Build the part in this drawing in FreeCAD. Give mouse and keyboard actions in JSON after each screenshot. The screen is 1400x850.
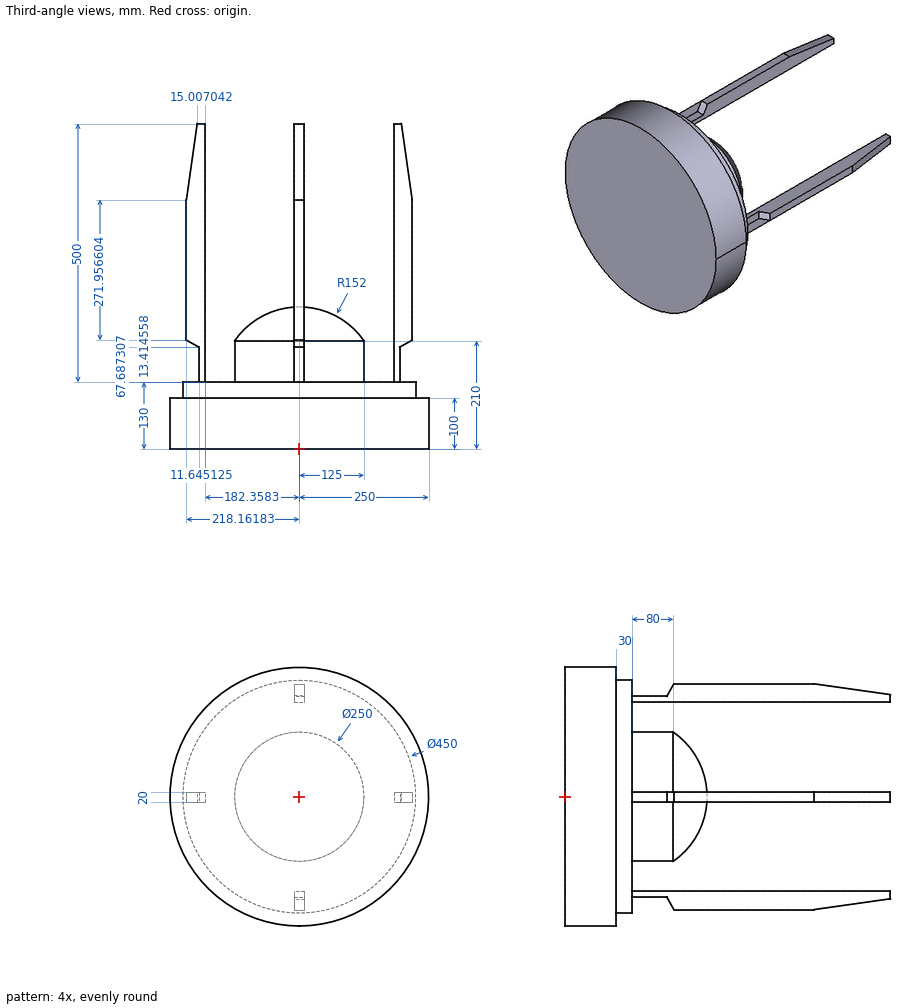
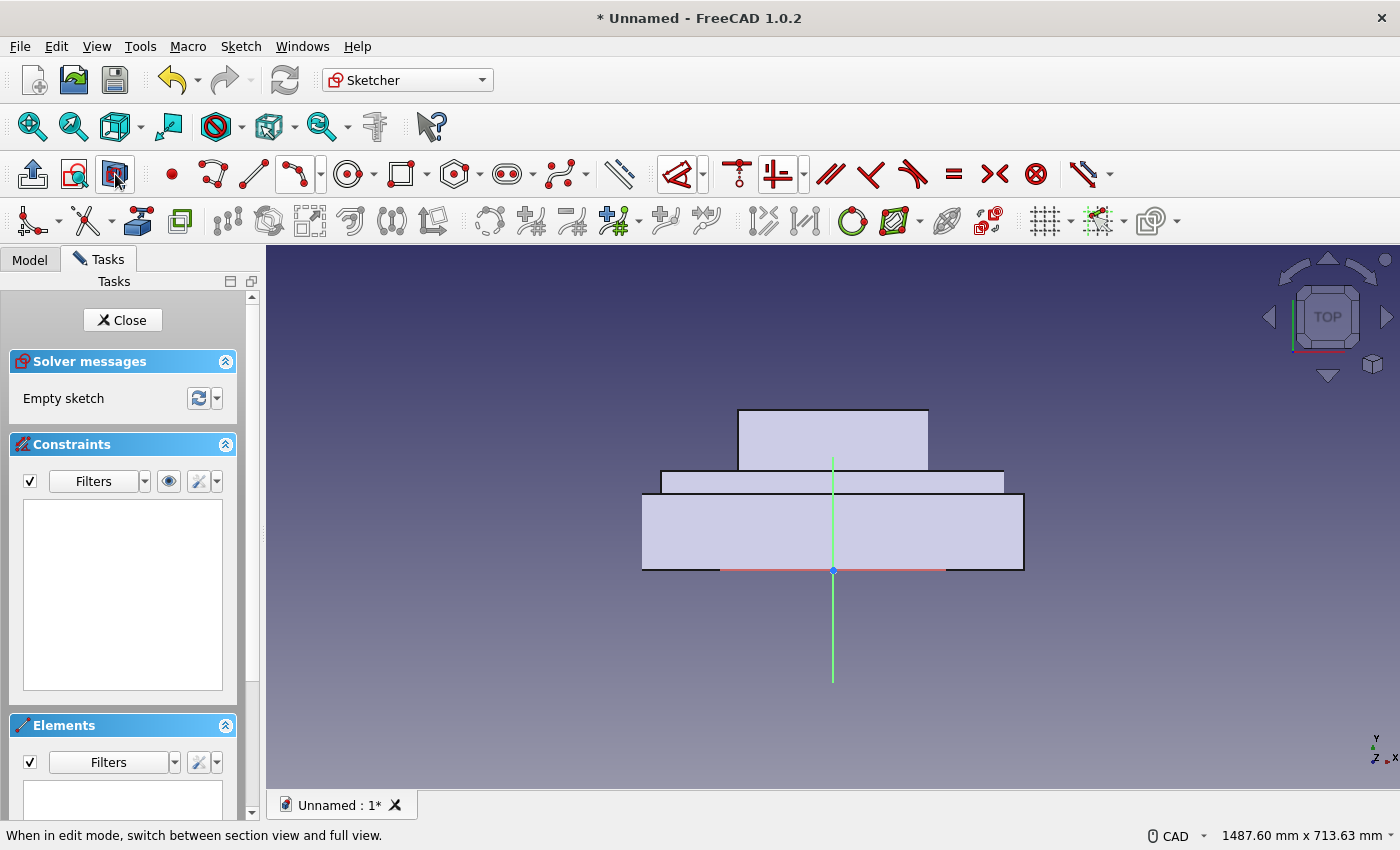
{"action": "scroll", "coordinate": [1117, 360], "scroll_direction": "up", "scroll_amount": 2}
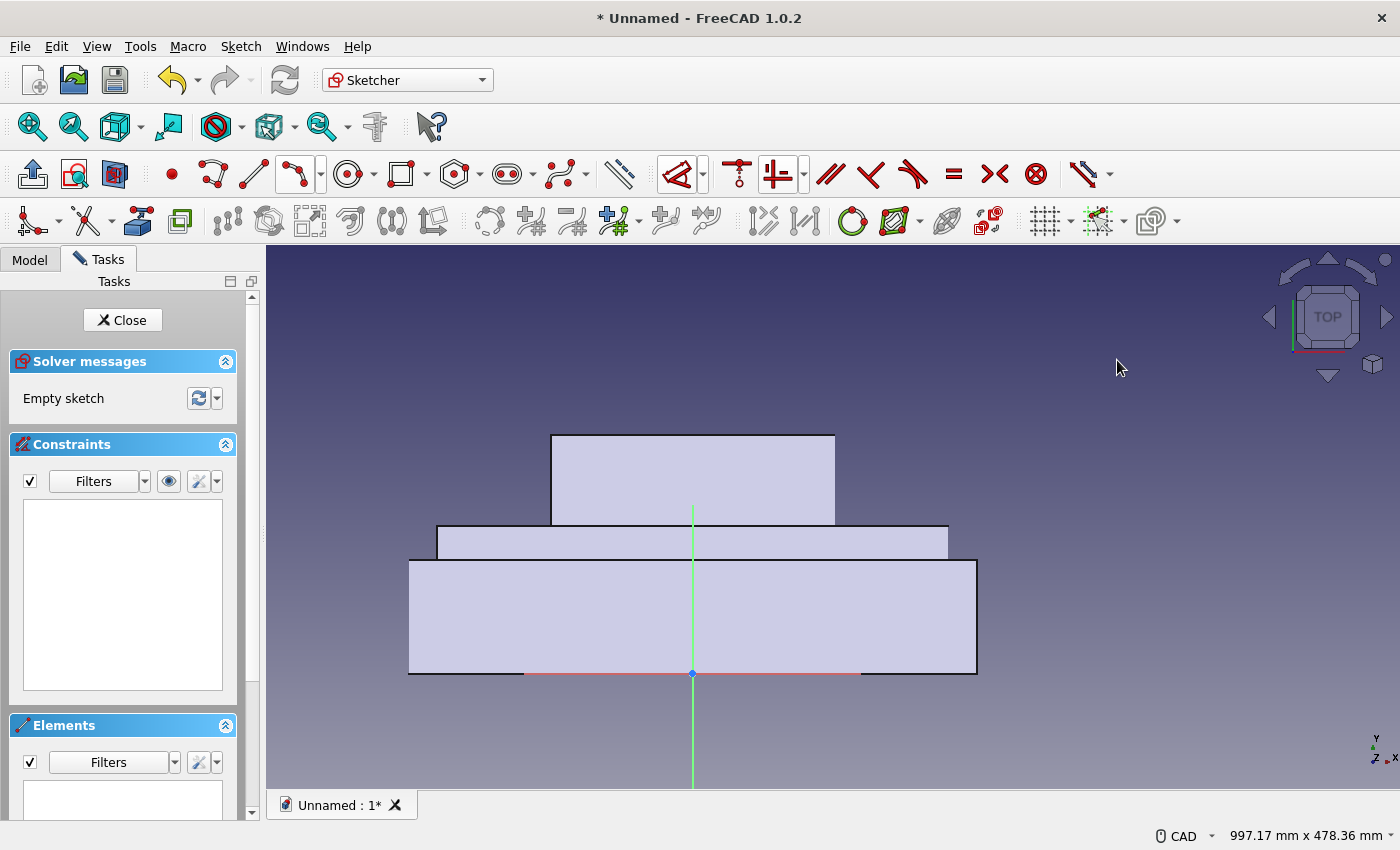
{"action": "left_click", "coordinate": [213, 174]}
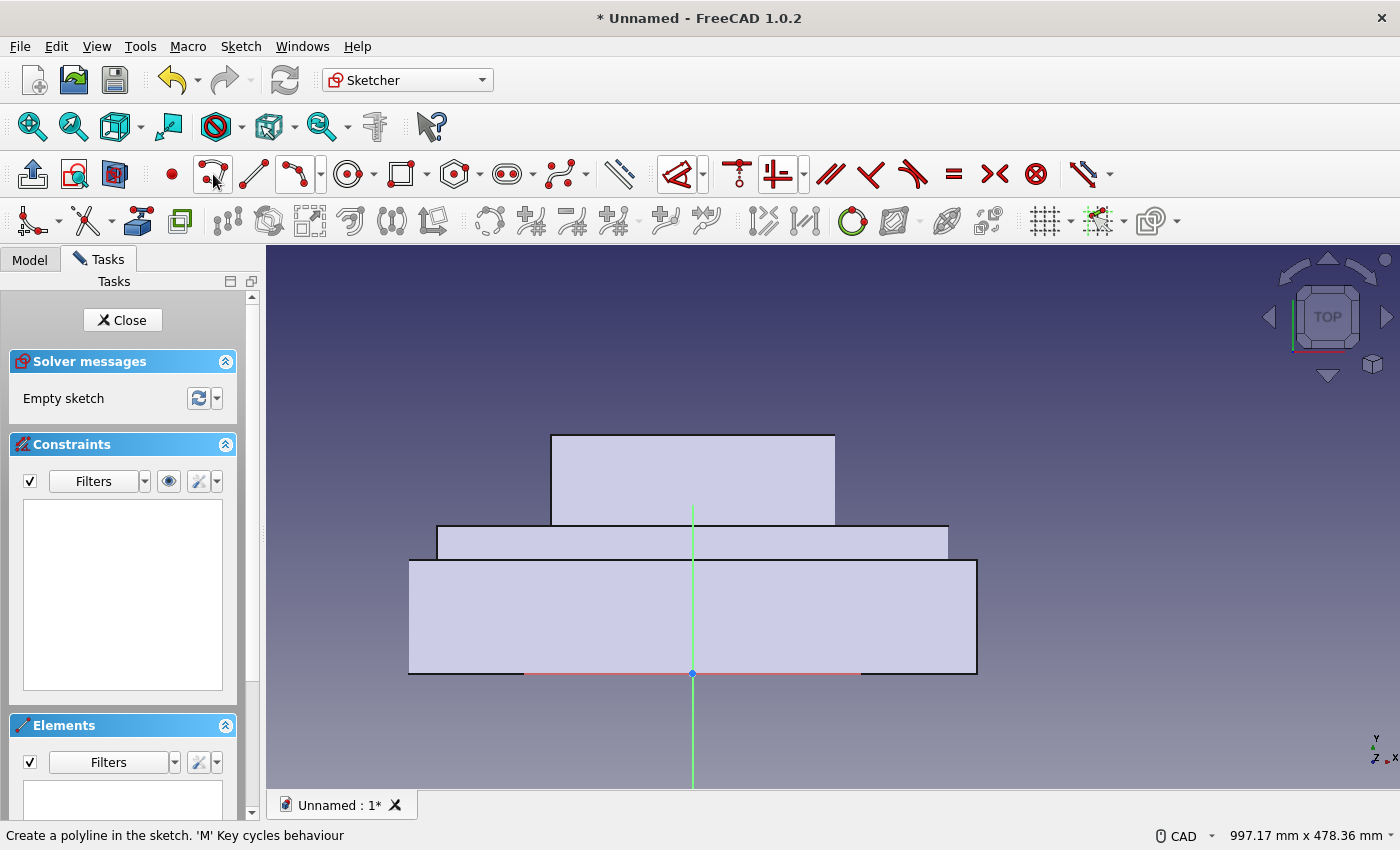
{"action": "left_click", "coordinate": [693, 360]}
{"action": "left_click", "coordinate": [702, 435]}
{"action": "left_click", "coordinate": [835, 435]}
{"action": "right_click", "coordinate": [835, 435]}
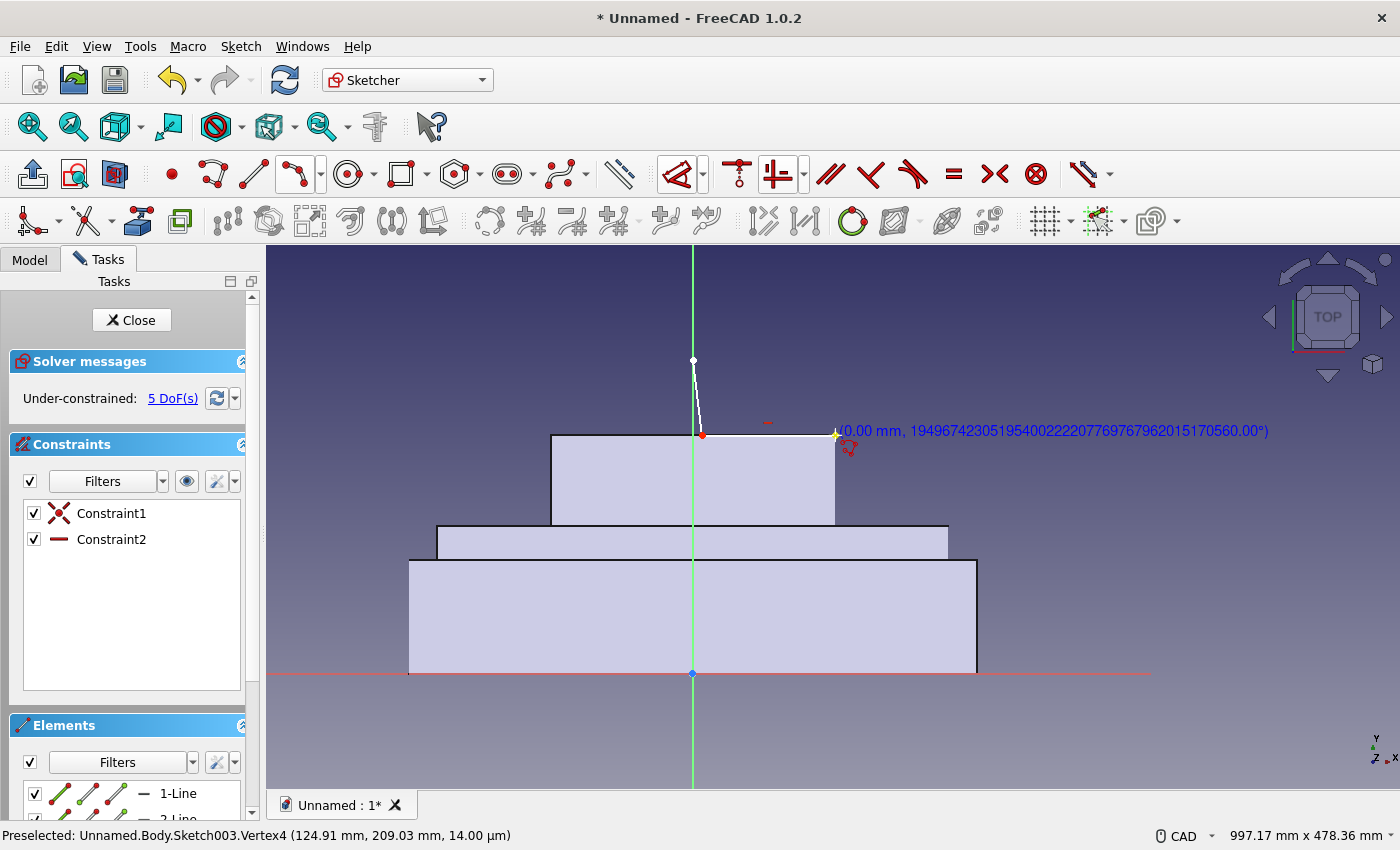
{"action": "left_click", "coordinate": [294, 174]}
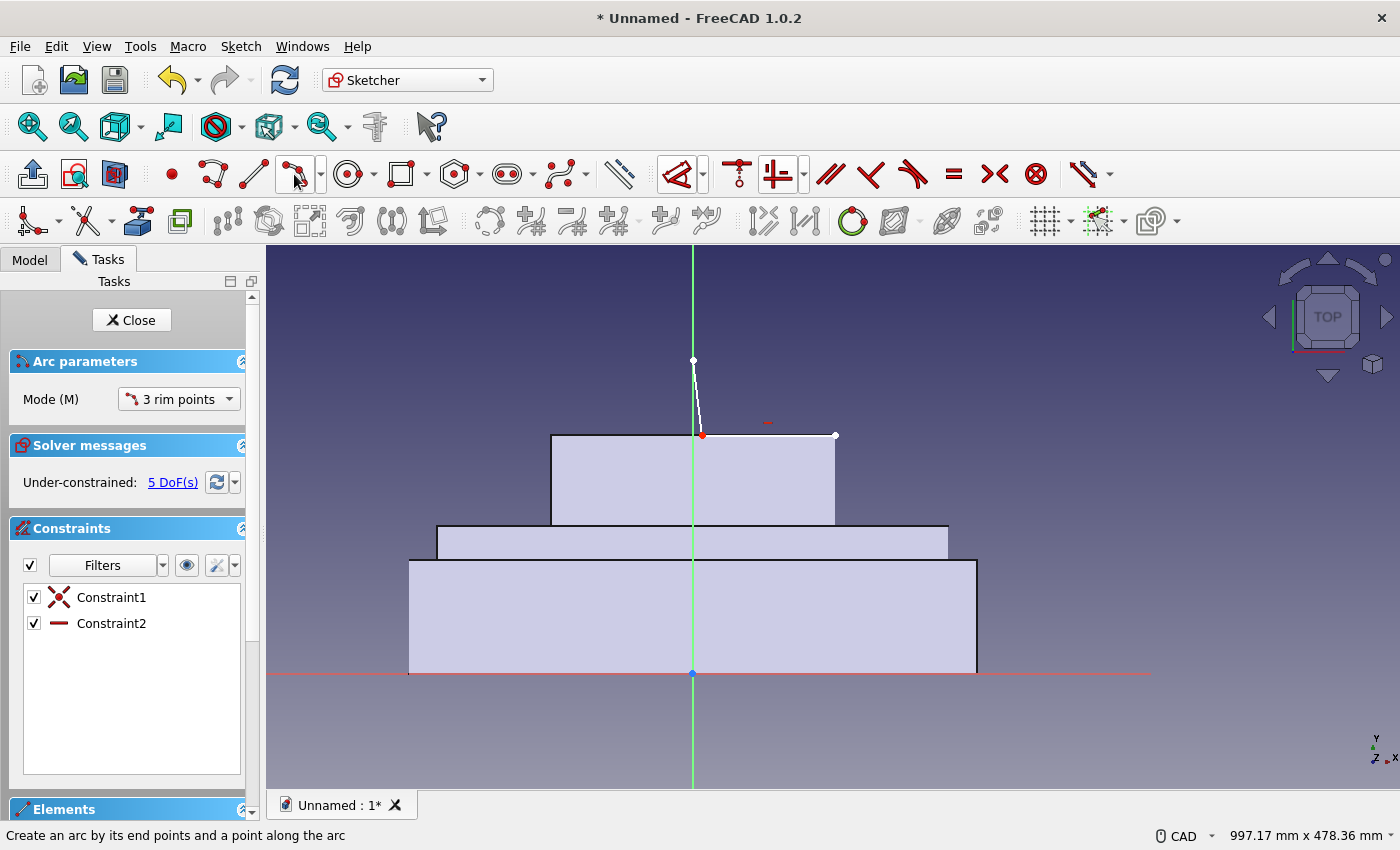
{"action": "left_click", "coordinate": [835, 436]}
{"action": "left_click", "coordinate": [693, 361]}
{"action": "left_click", "coordinate": [773, 380]}
{"action": "key", "text": "Escape"}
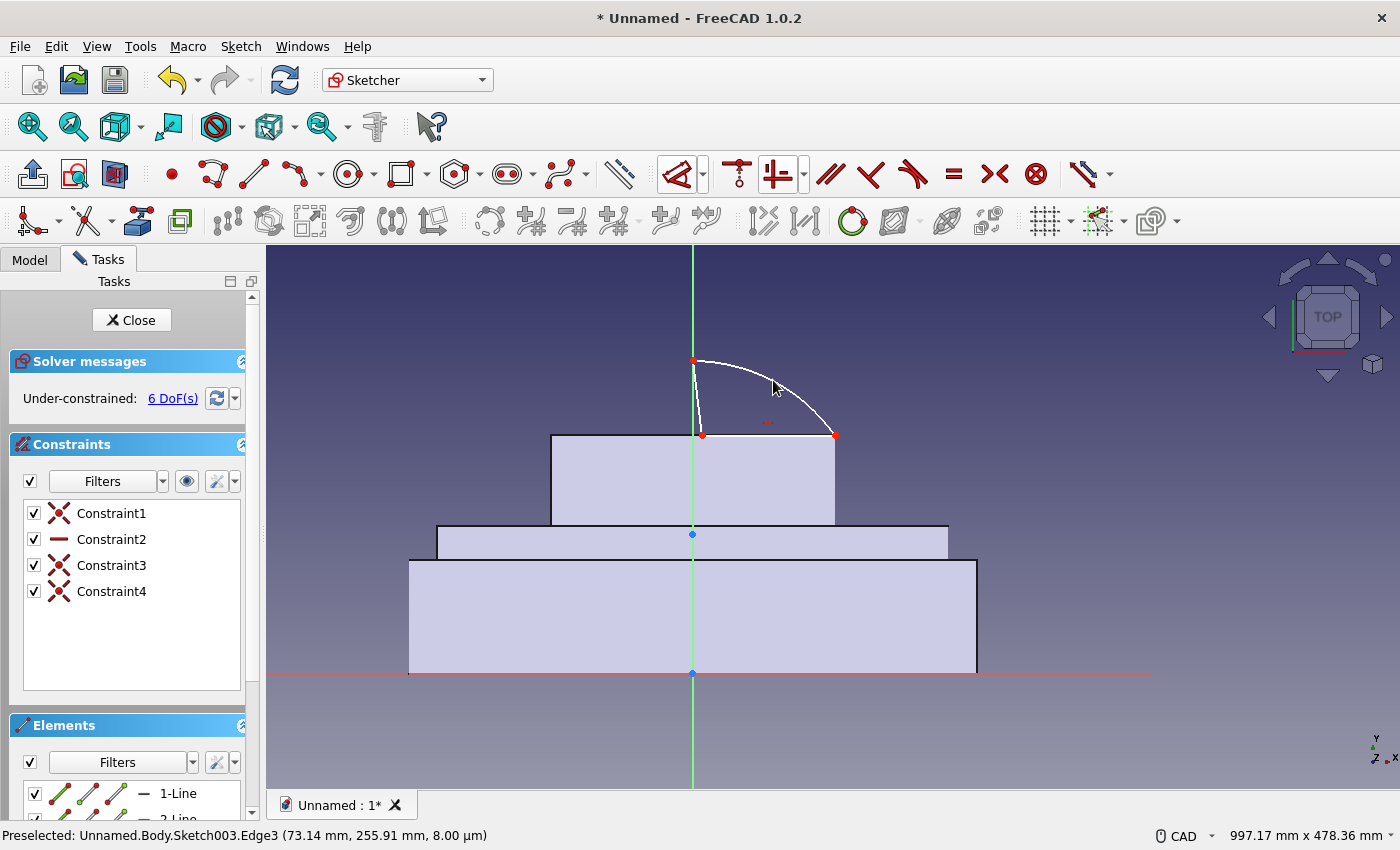
{"action": "left_click", "coordinate": [696, 383]}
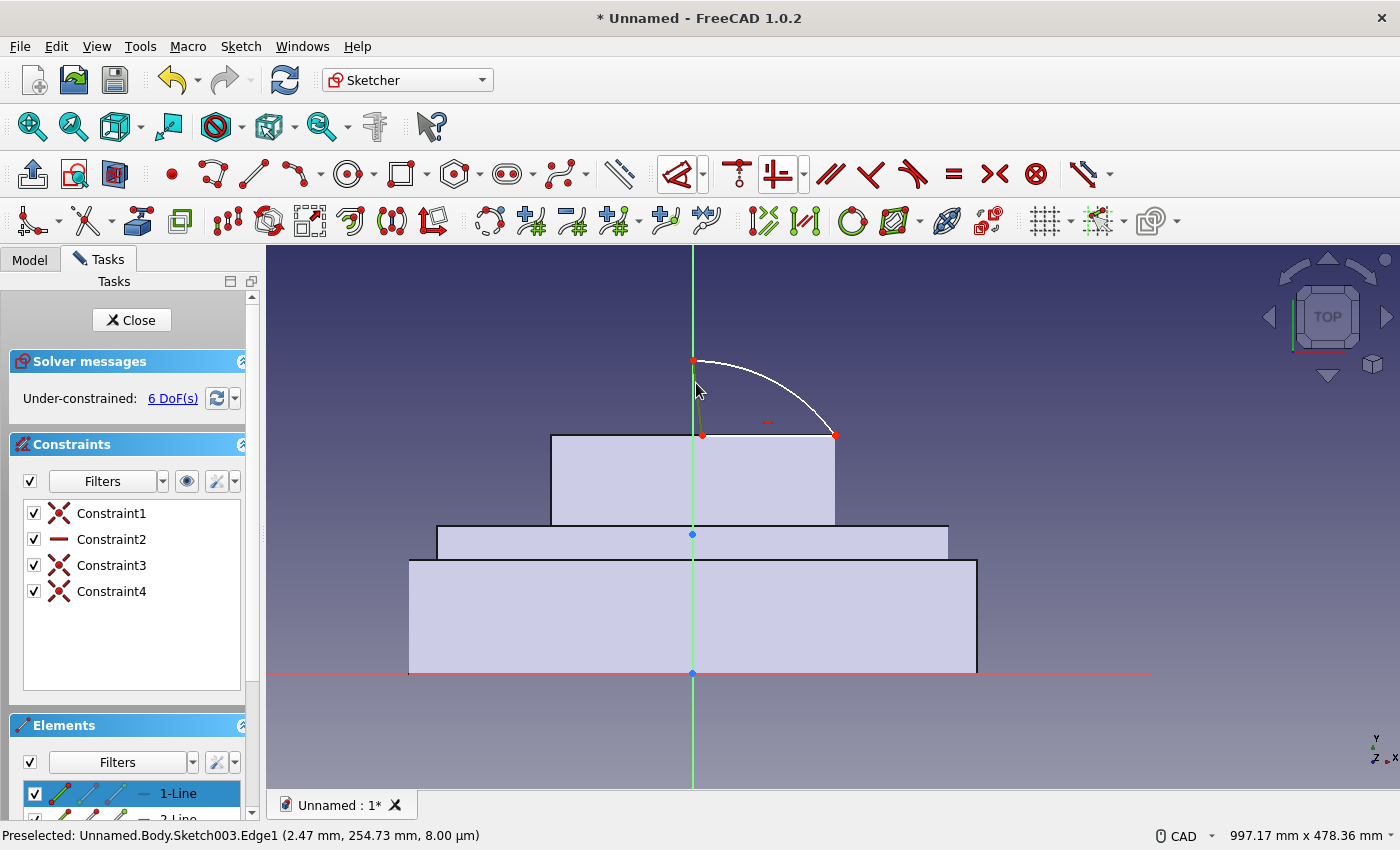
{"action": "left_click", "coordinate": [804, 174]}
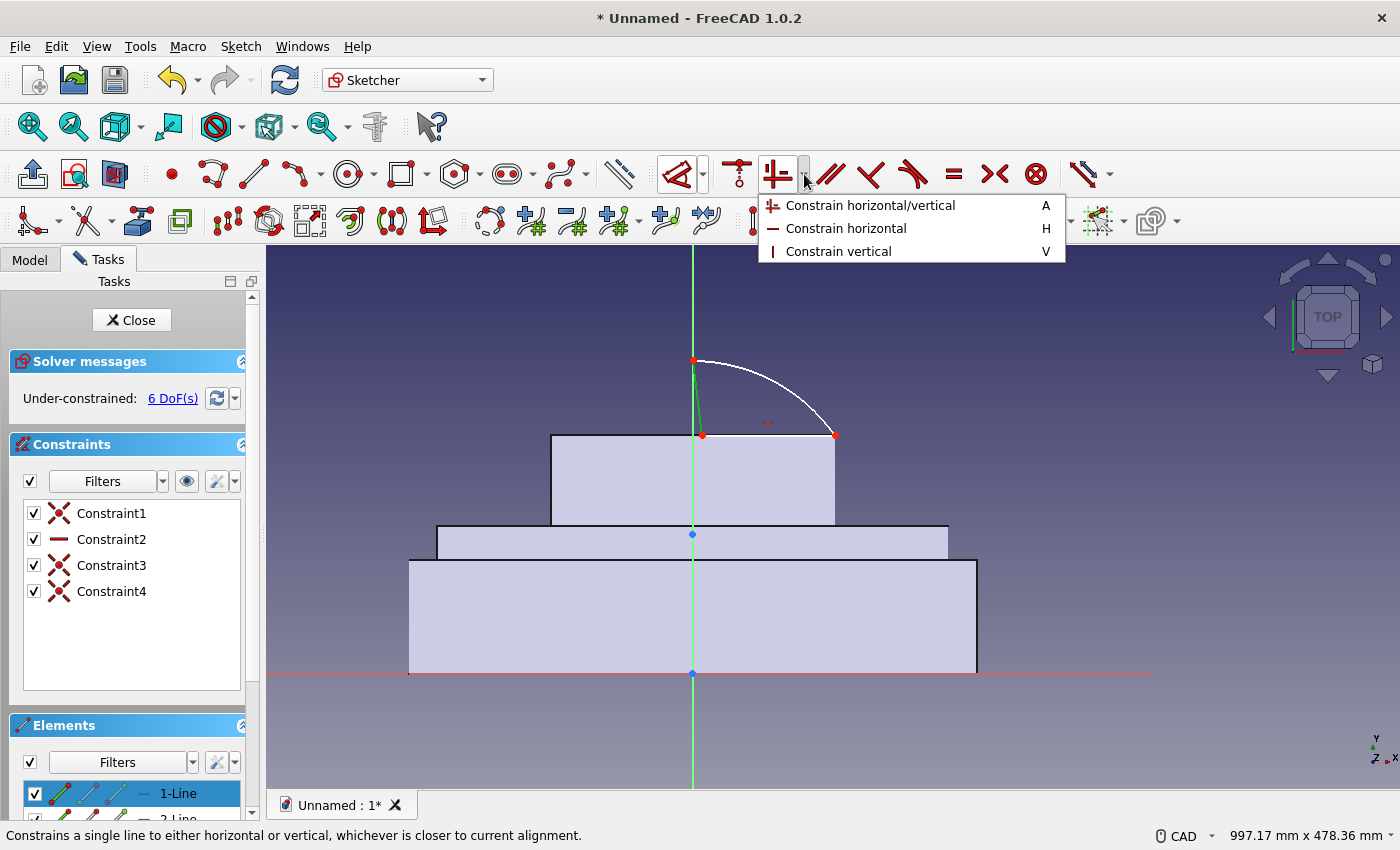
{"action": "left_click", "coordinate": [912, 252]}